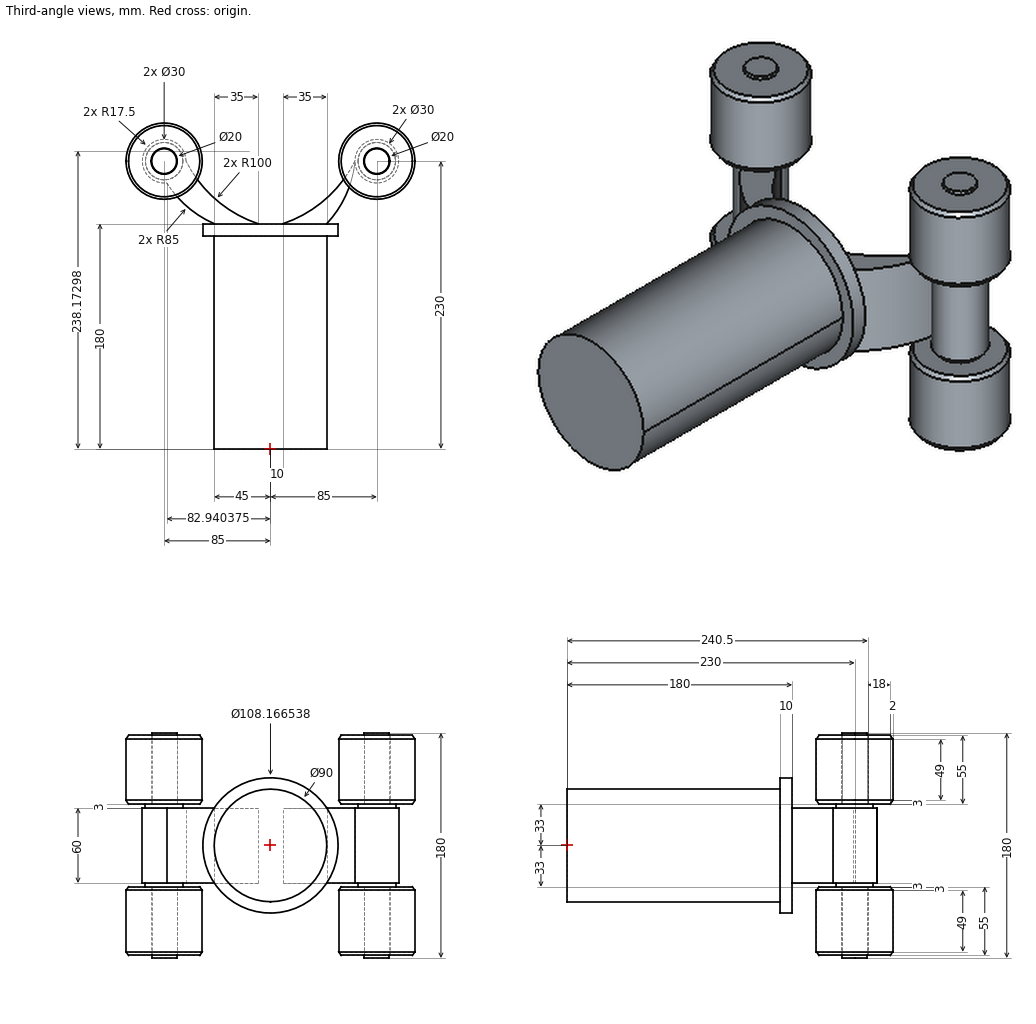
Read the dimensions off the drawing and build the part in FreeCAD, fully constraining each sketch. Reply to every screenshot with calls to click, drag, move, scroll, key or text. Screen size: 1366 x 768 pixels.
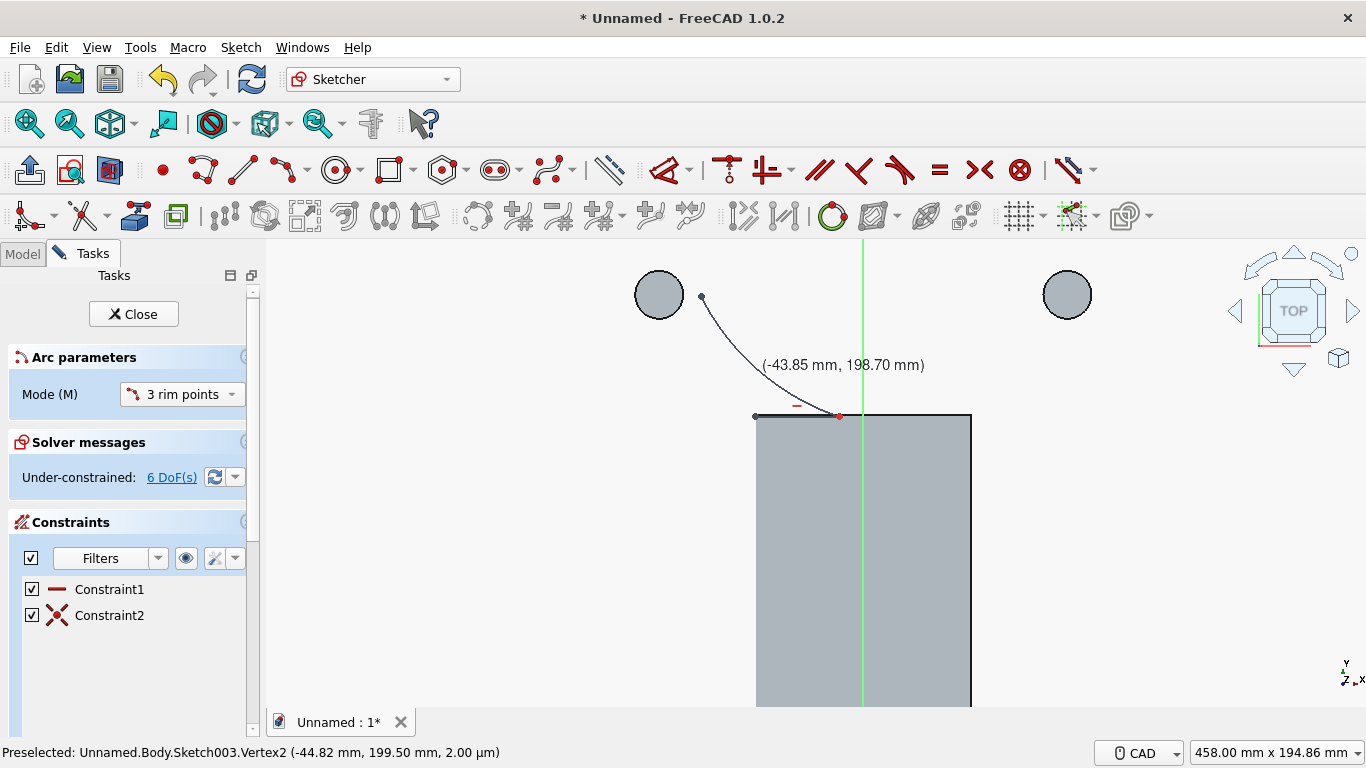
click(701, 297)
click(664, 337)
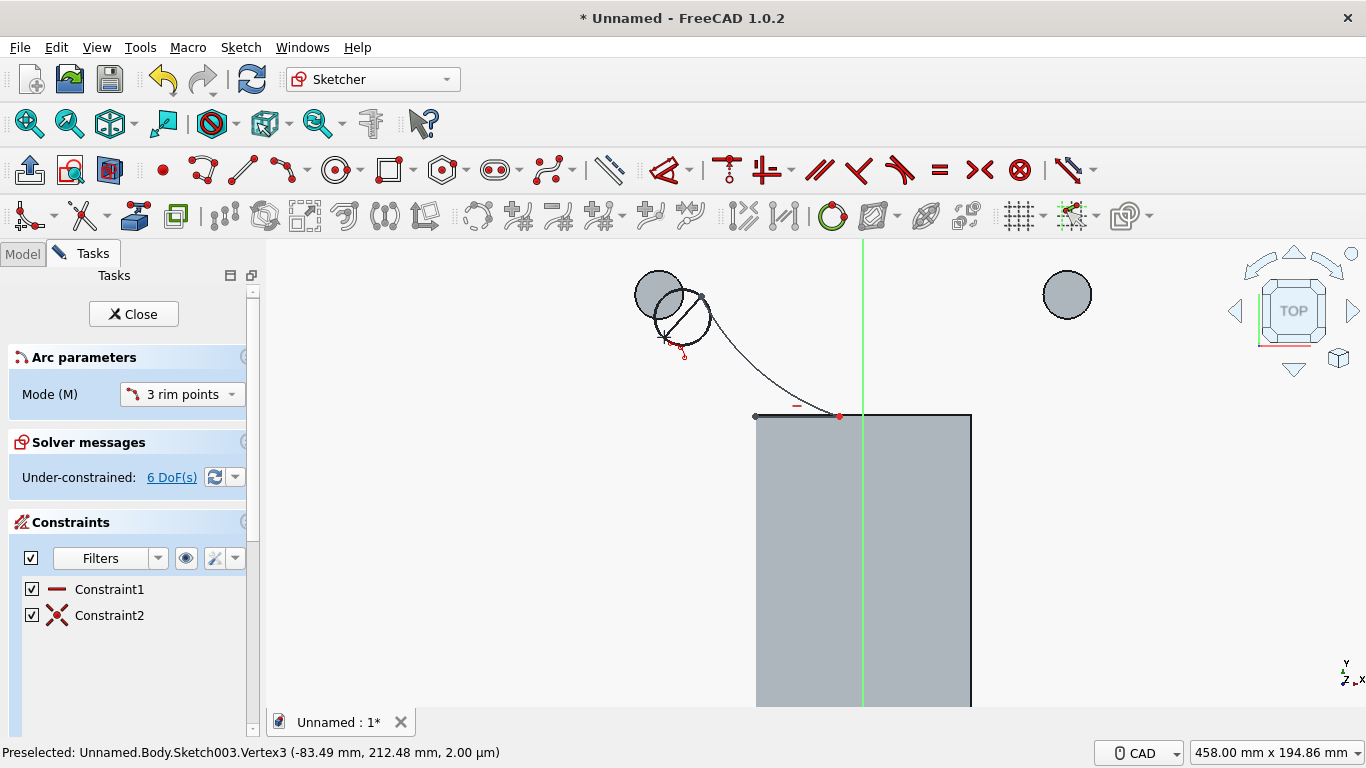
scroll(600, 371, down, 3)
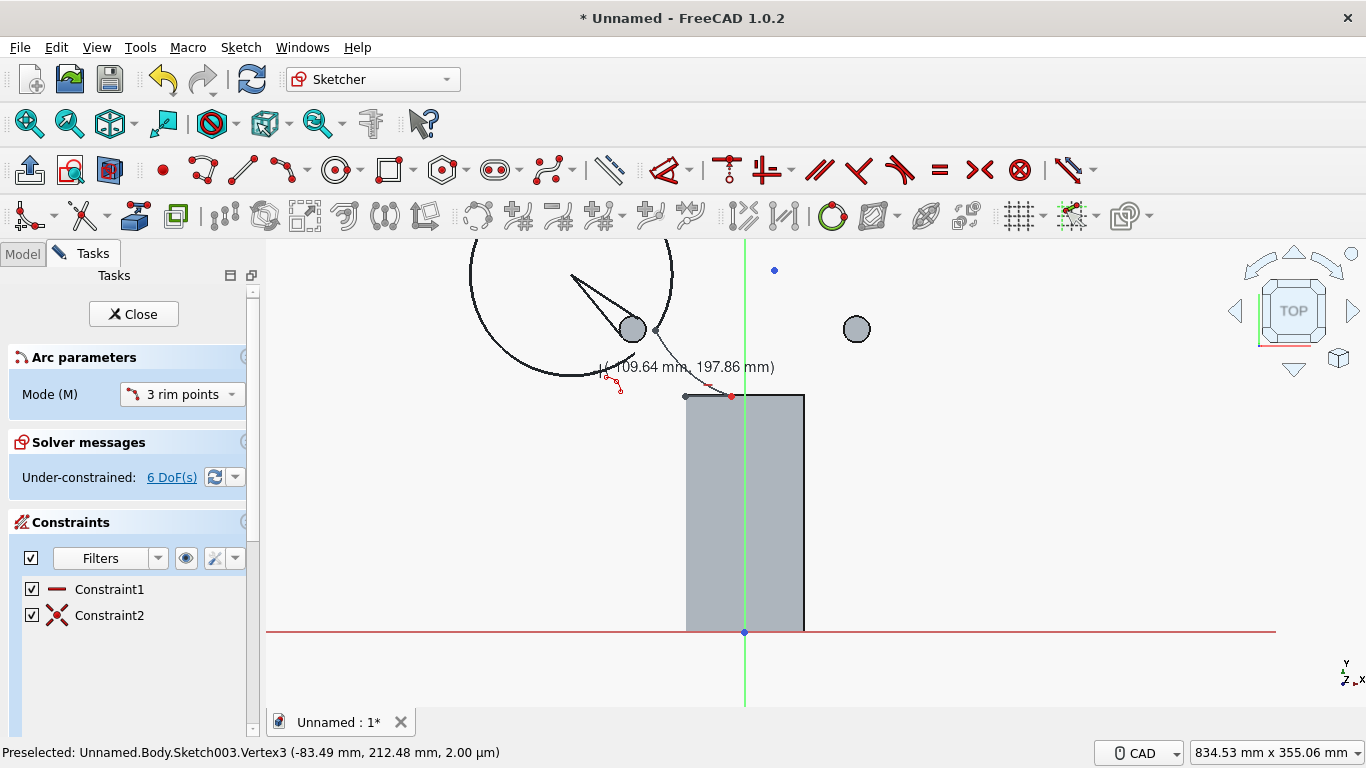
click(615, 314)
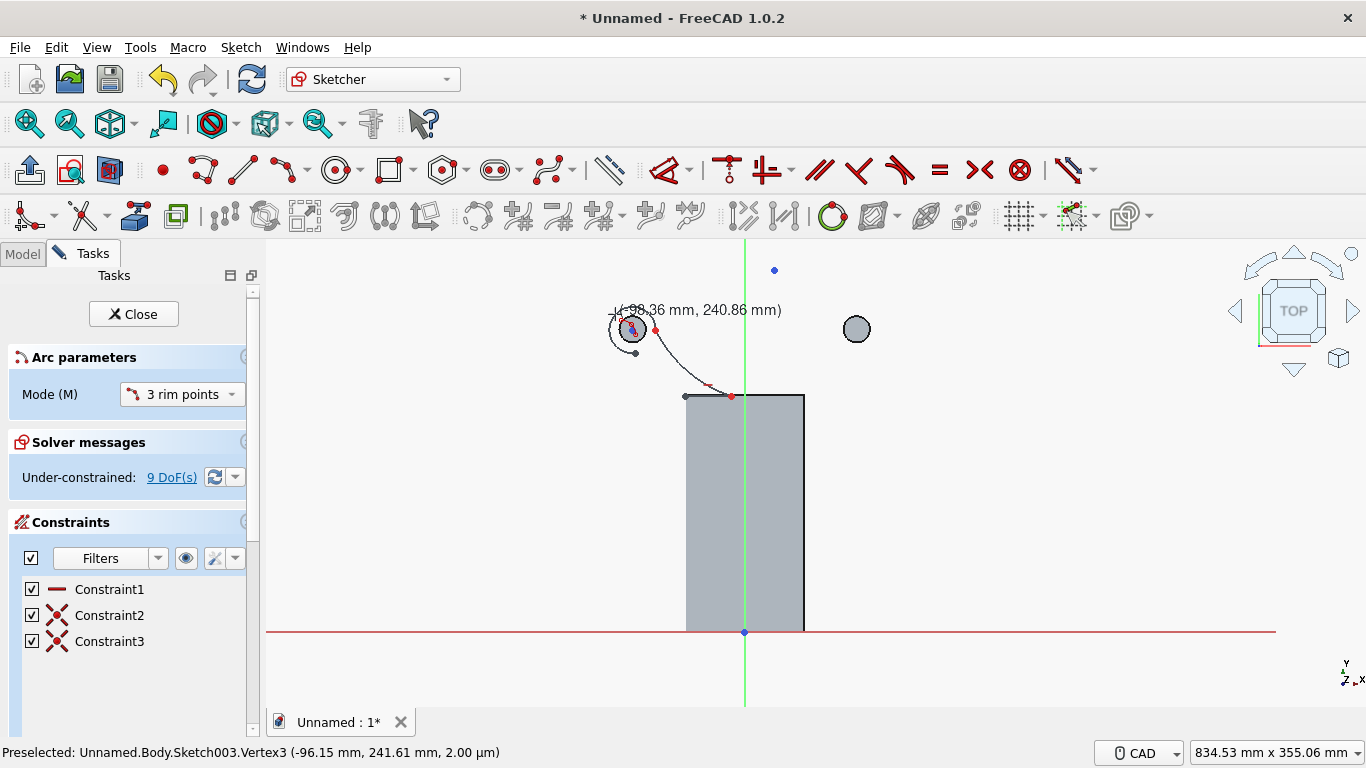
click(635, 353)
click(686, 396)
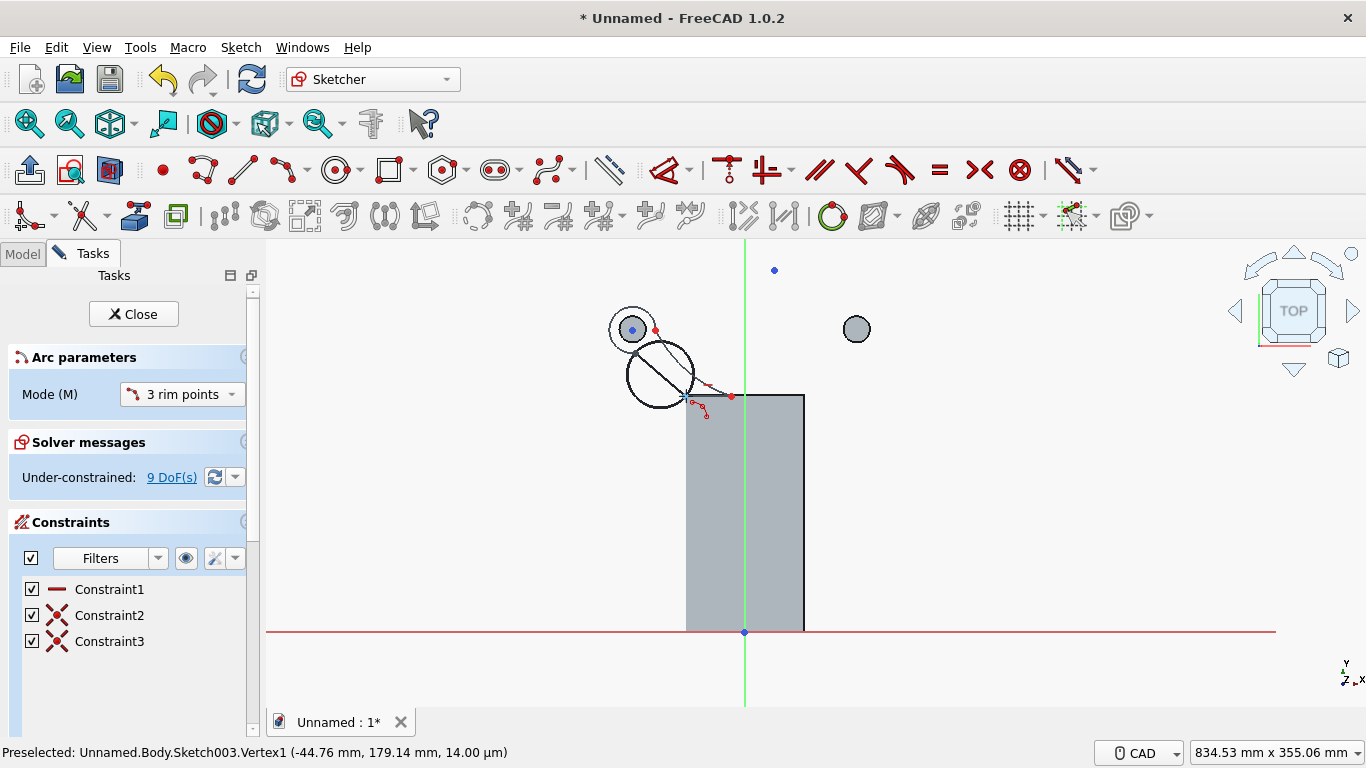
scroll(657, 377, up, 6)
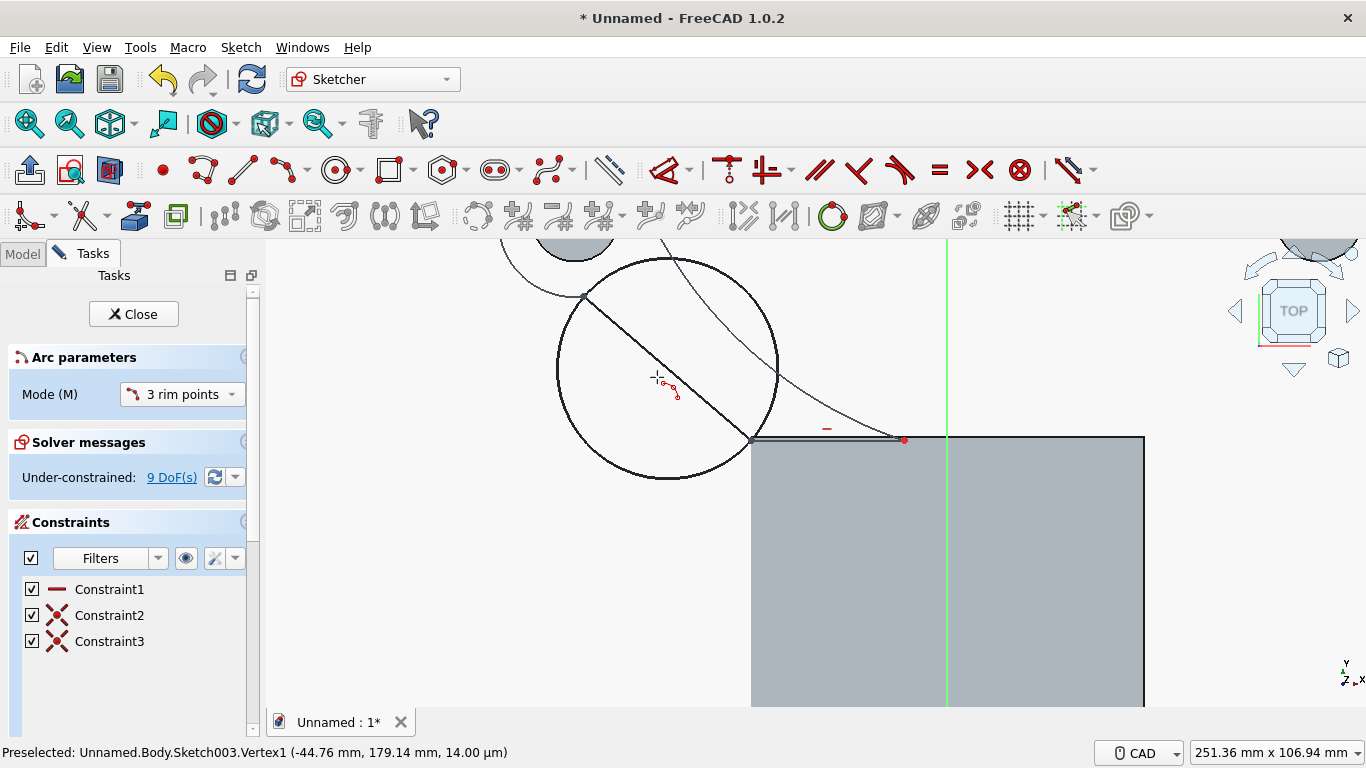
click(656, 378)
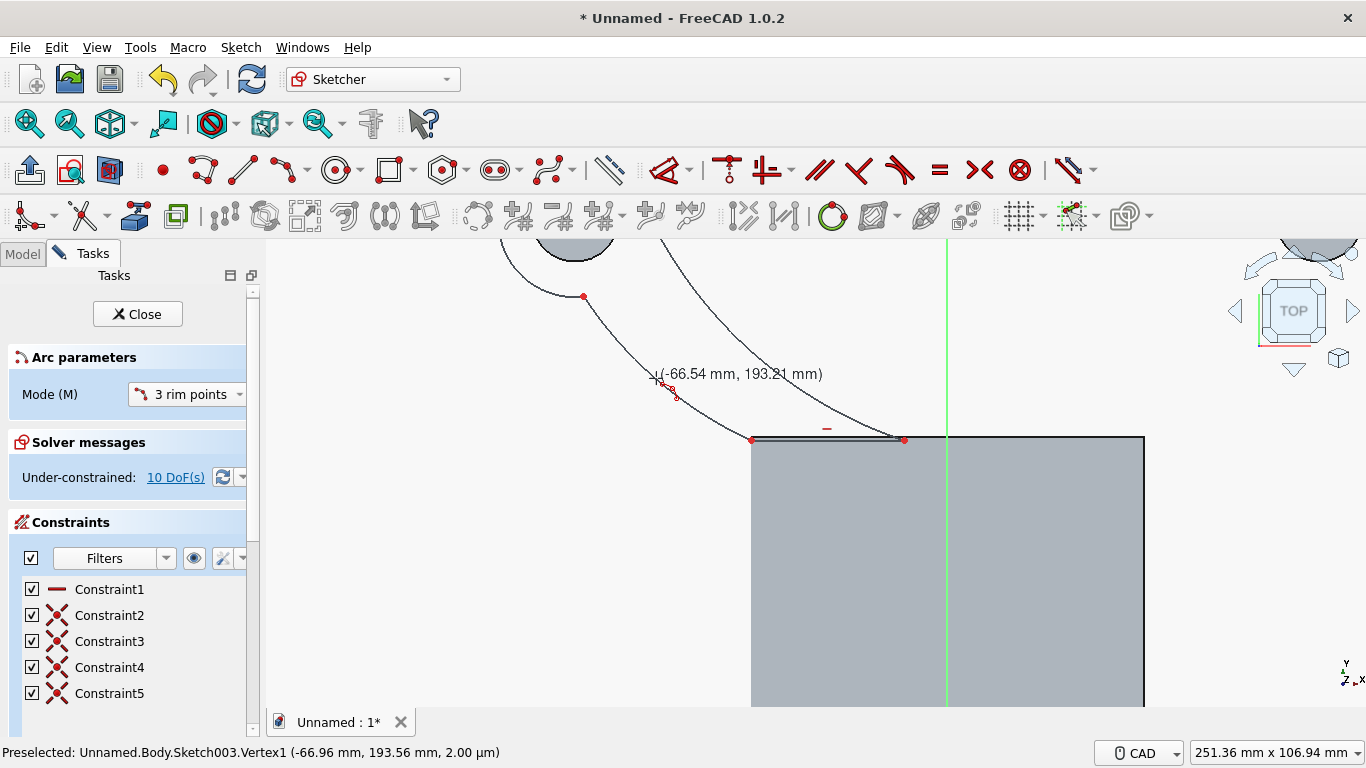
click(244, 170)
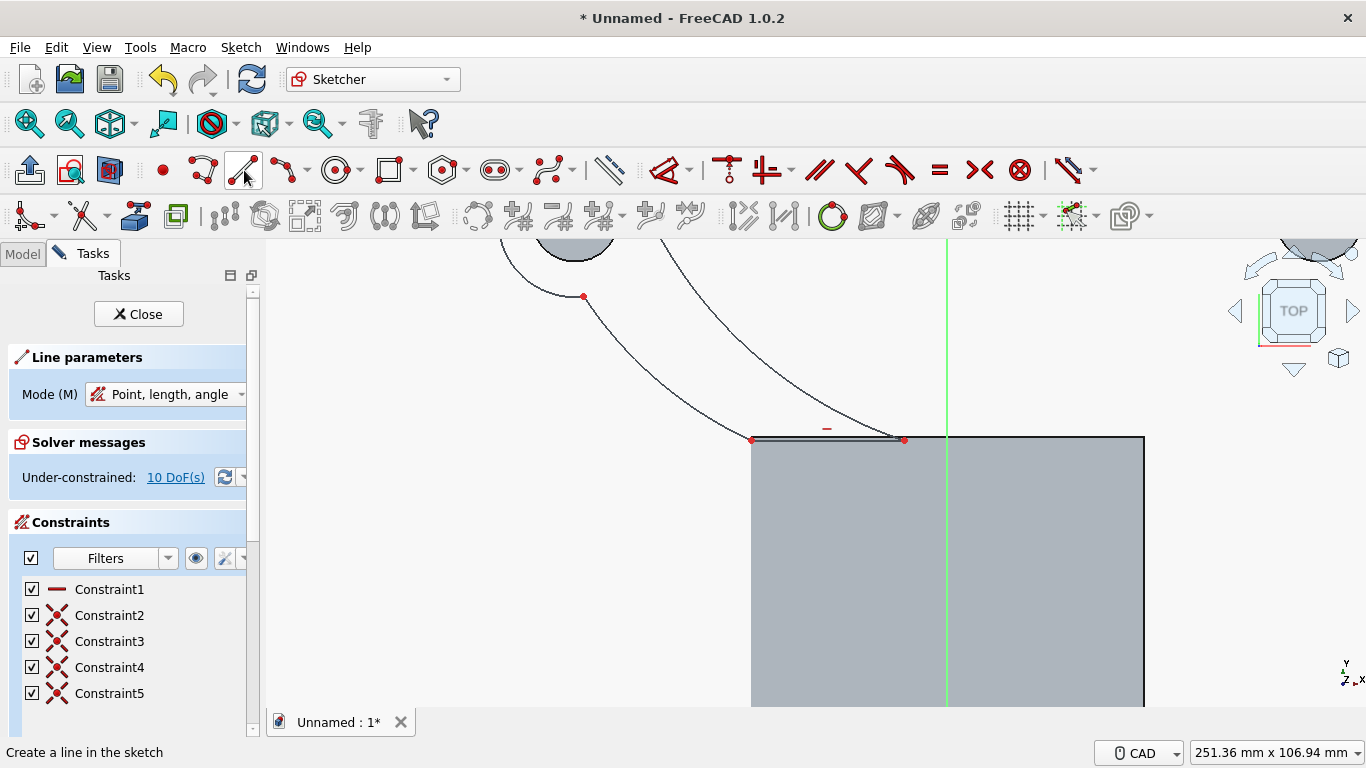
click(991, 437)
click(1144, 437)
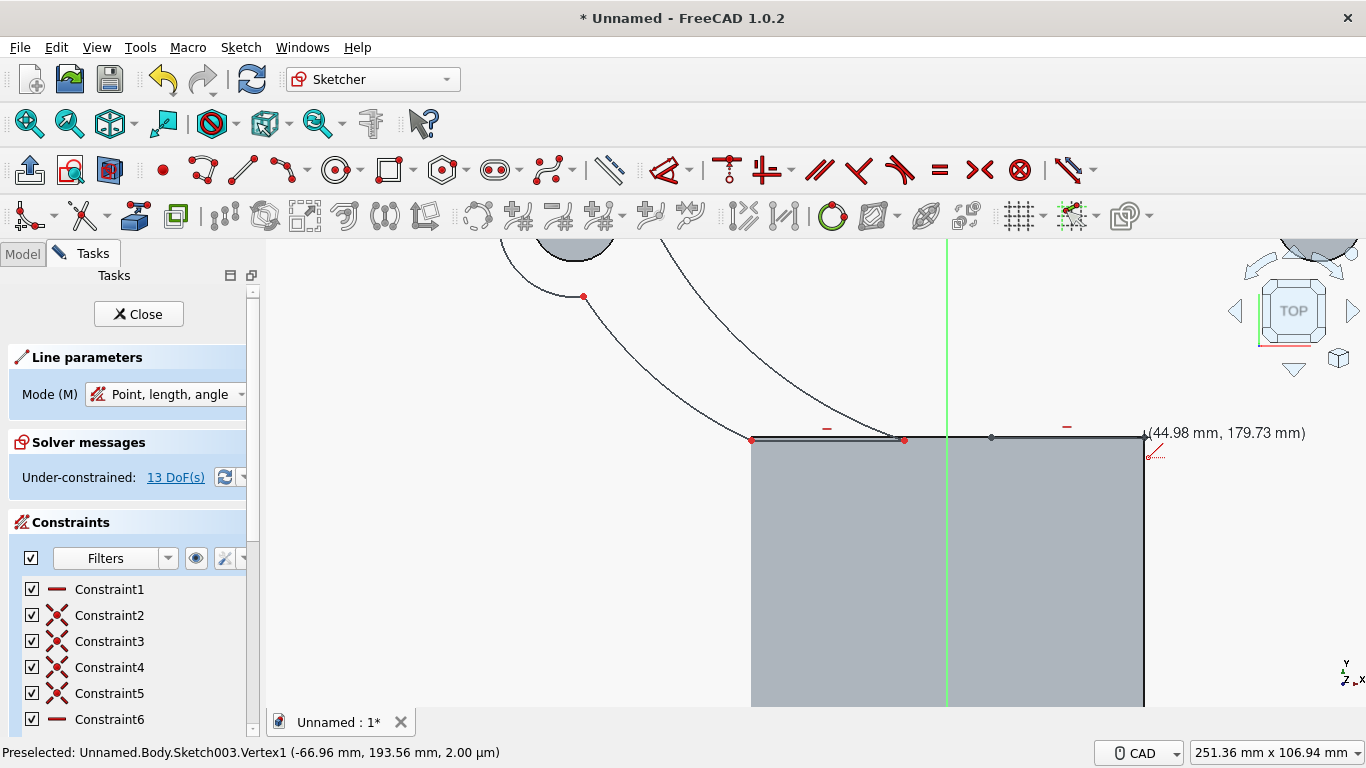
click(284, 170)